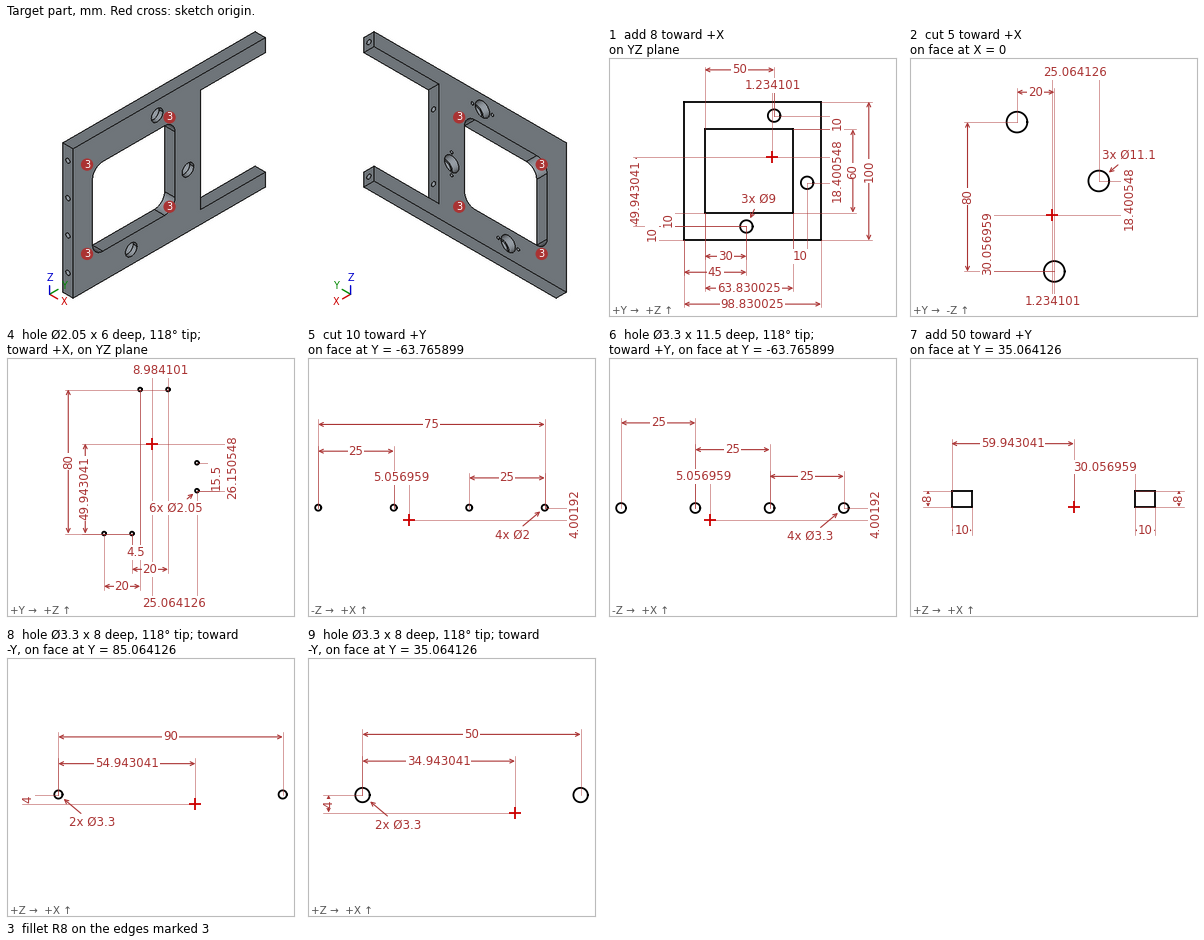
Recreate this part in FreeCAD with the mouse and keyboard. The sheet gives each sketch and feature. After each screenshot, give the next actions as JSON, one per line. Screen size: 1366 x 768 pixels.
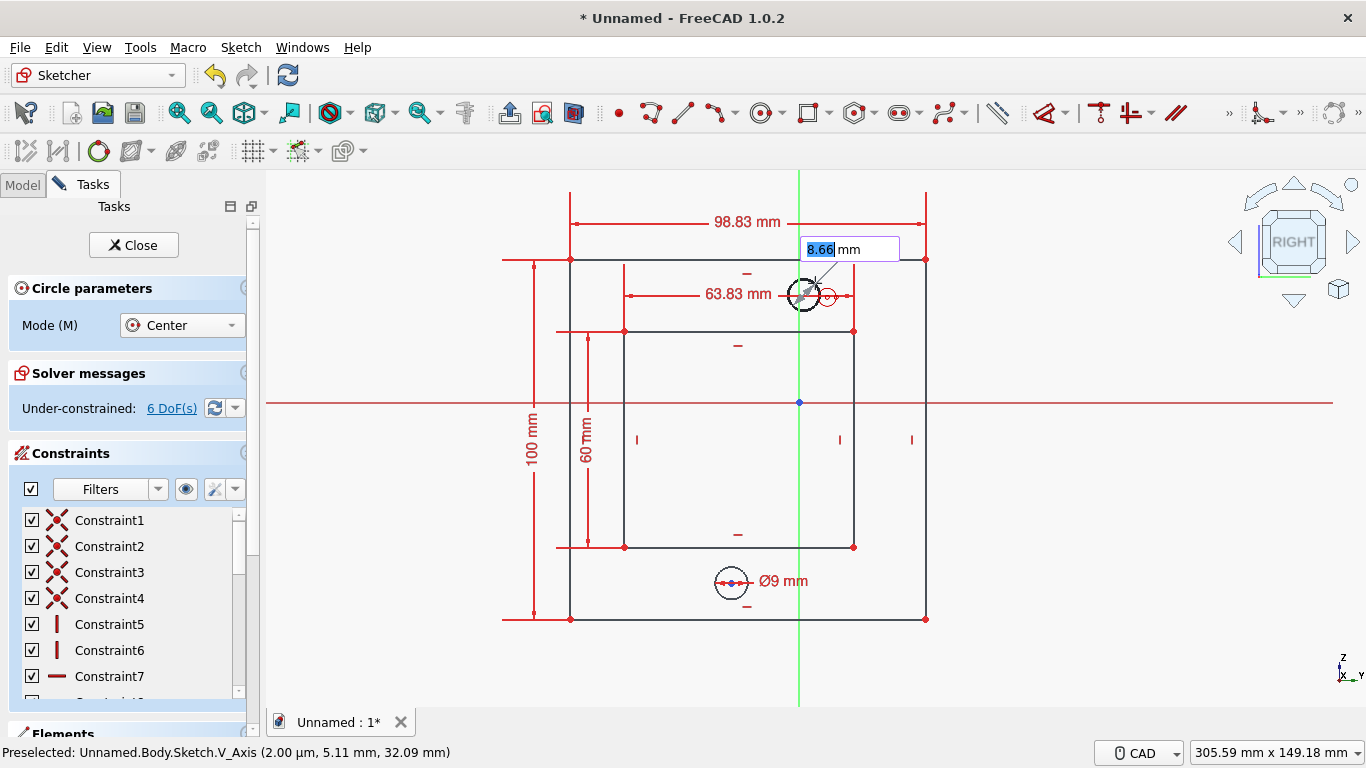
{"action": "type", "text": "9"}
{"action": "key", "text": "Return"}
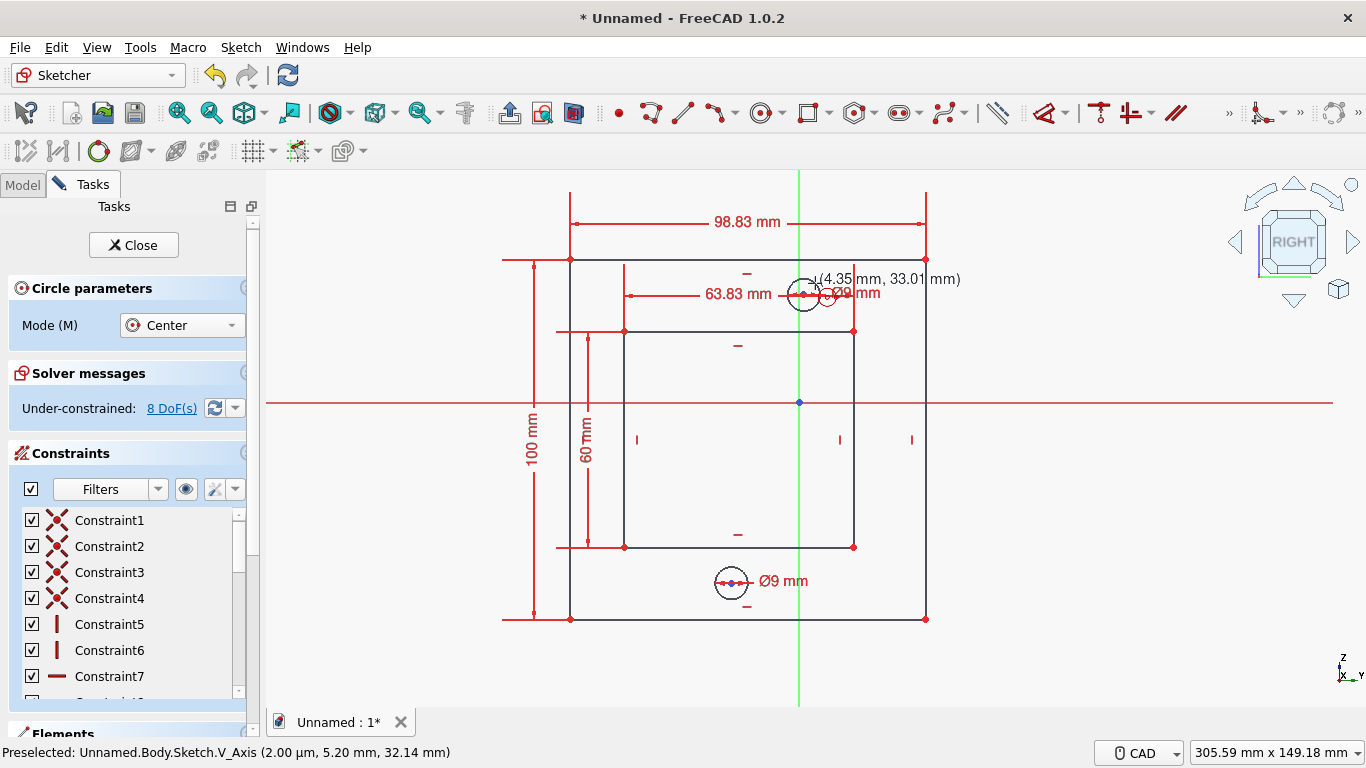
{"action": "scroll", "coordinate": [890, 469], "scroll_direction": "up", "scroll_amount": 2}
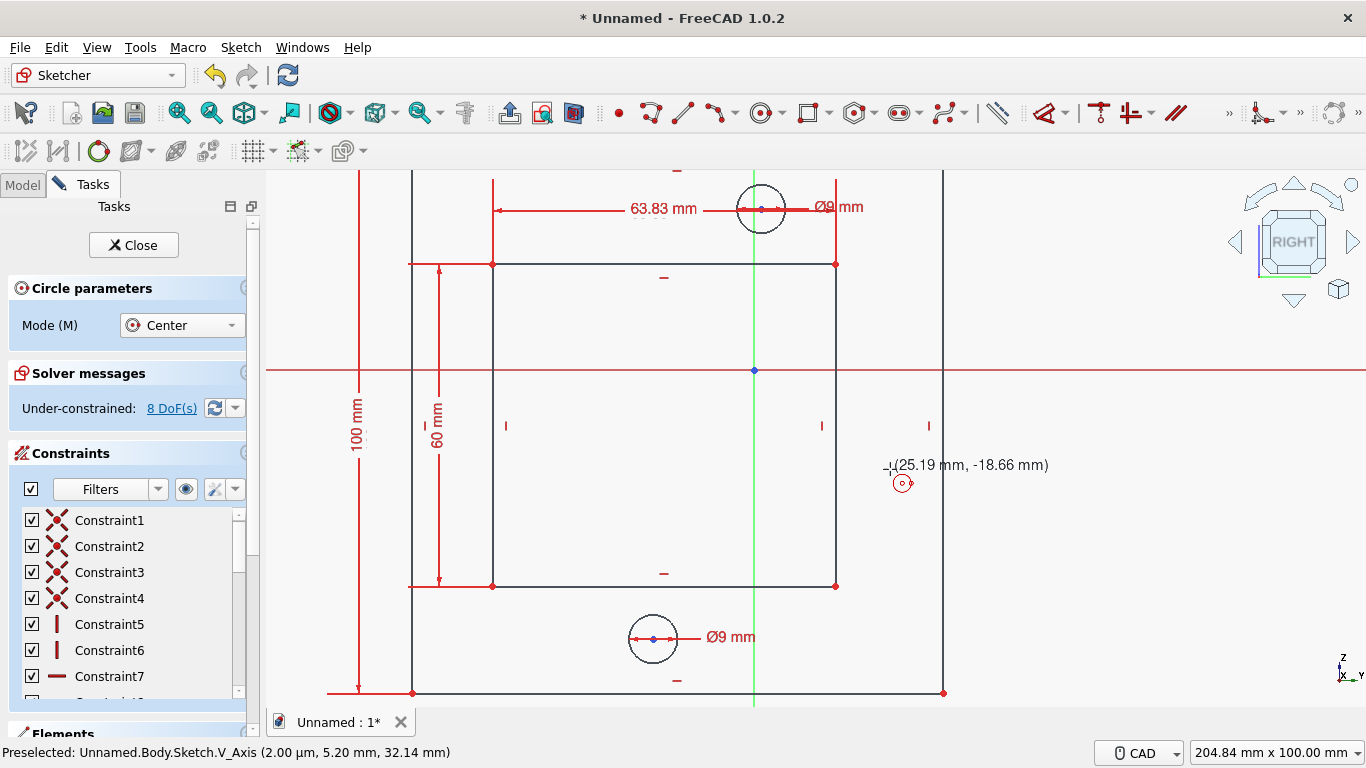
{"action": "left_click", "coordinate": [889, 469]}
{"action": "mouse_move", "coordinate": [906, 452]}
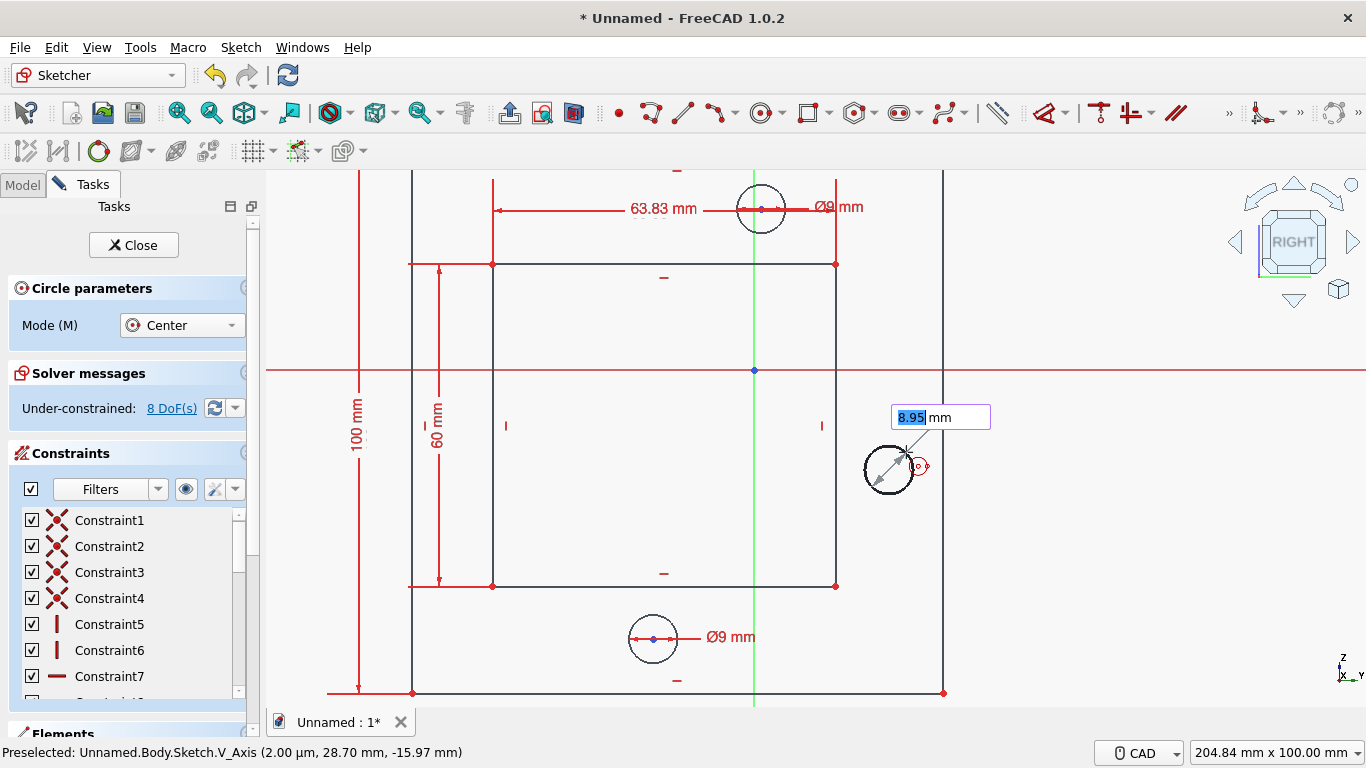
{"action": "type", "text": "9"}
{"action": "key", "text": "Return"}
{"action": "key", "text": "Escape"}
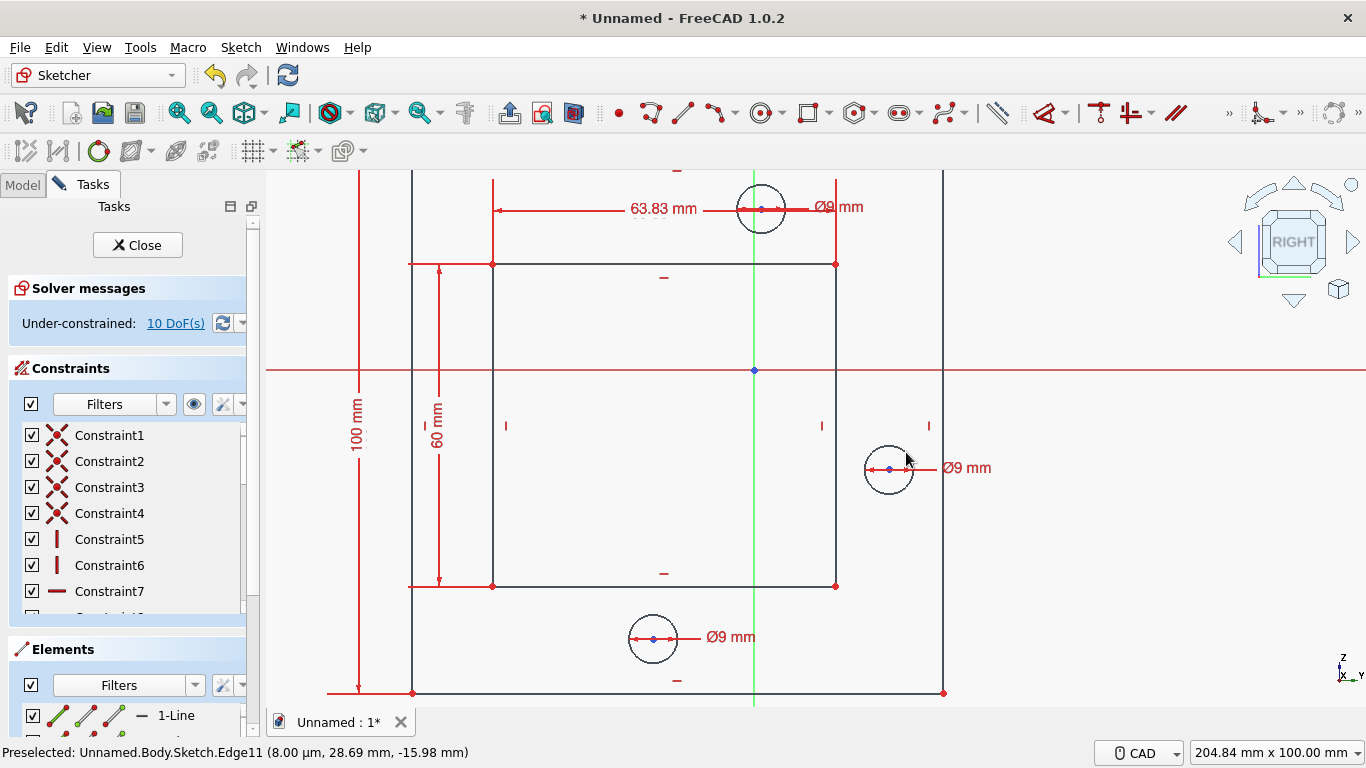
{"action": "left_click", "coordinate": [493, 587]}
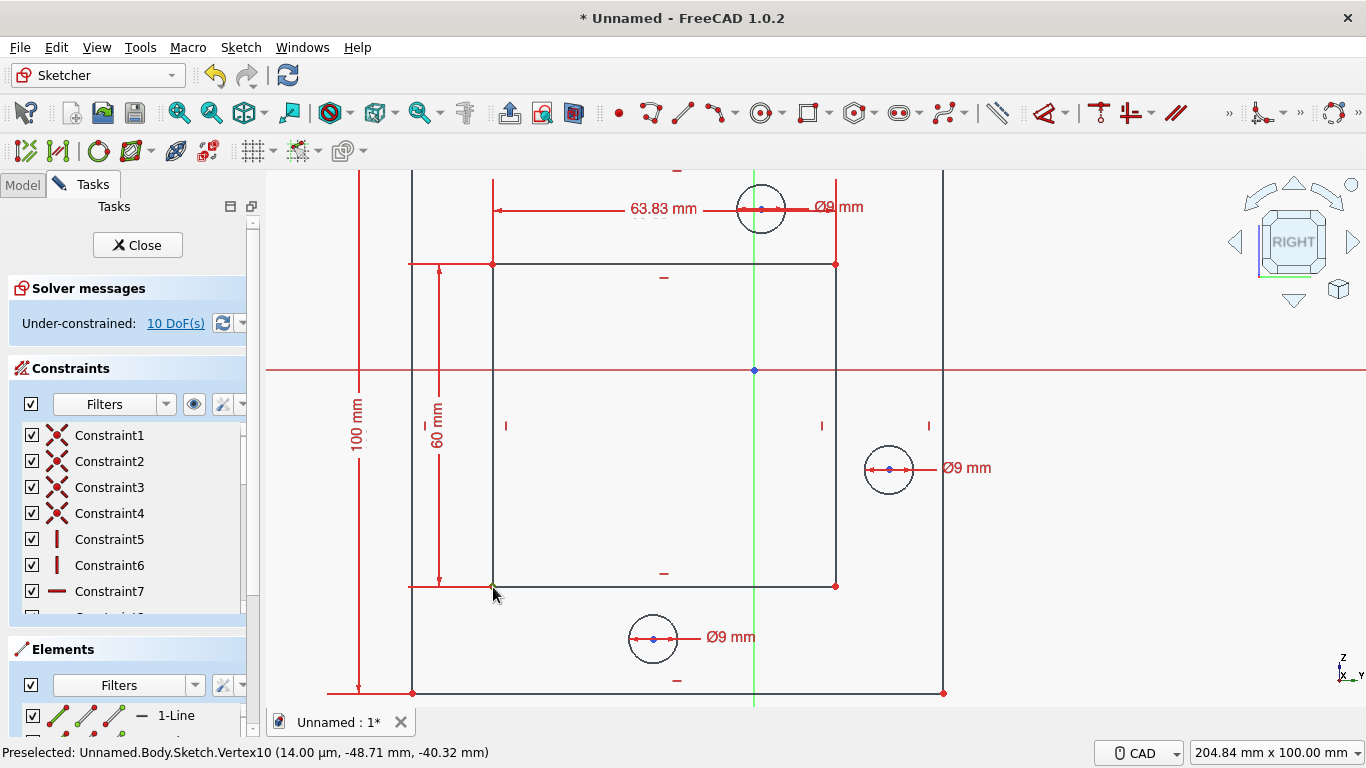
{"action": "left_click", "coordinate": [653, 639]}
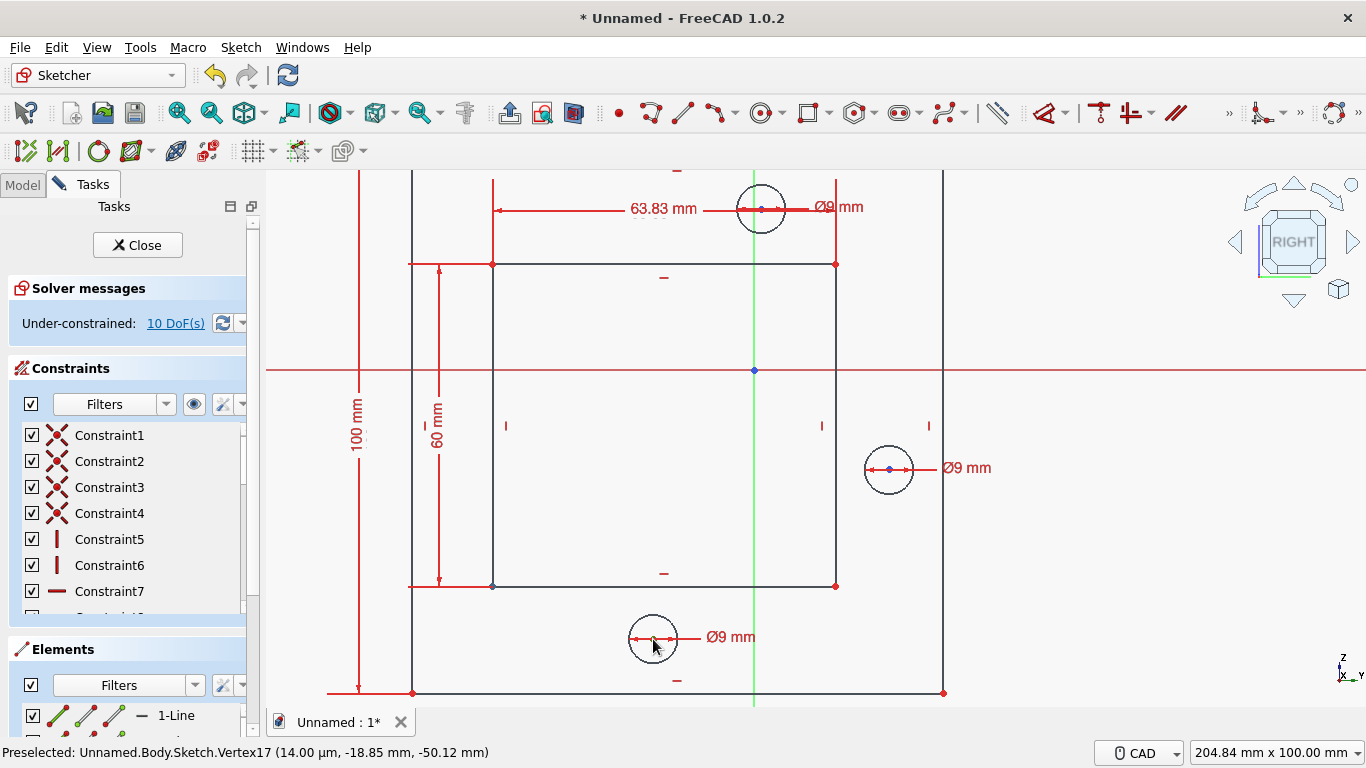
{"action": "key", "text": "l"}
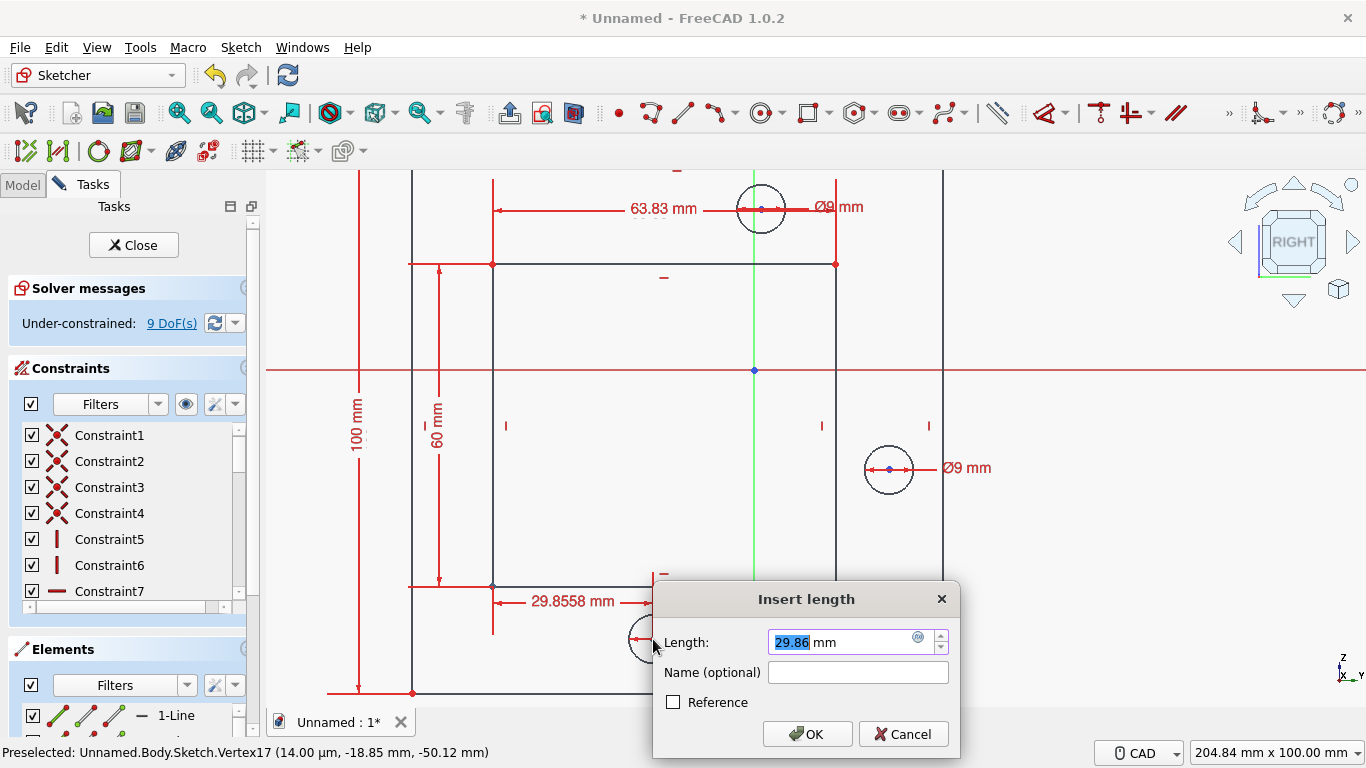
{"action": "type", "text": "30"}
{"action": "key", "text": "Return"}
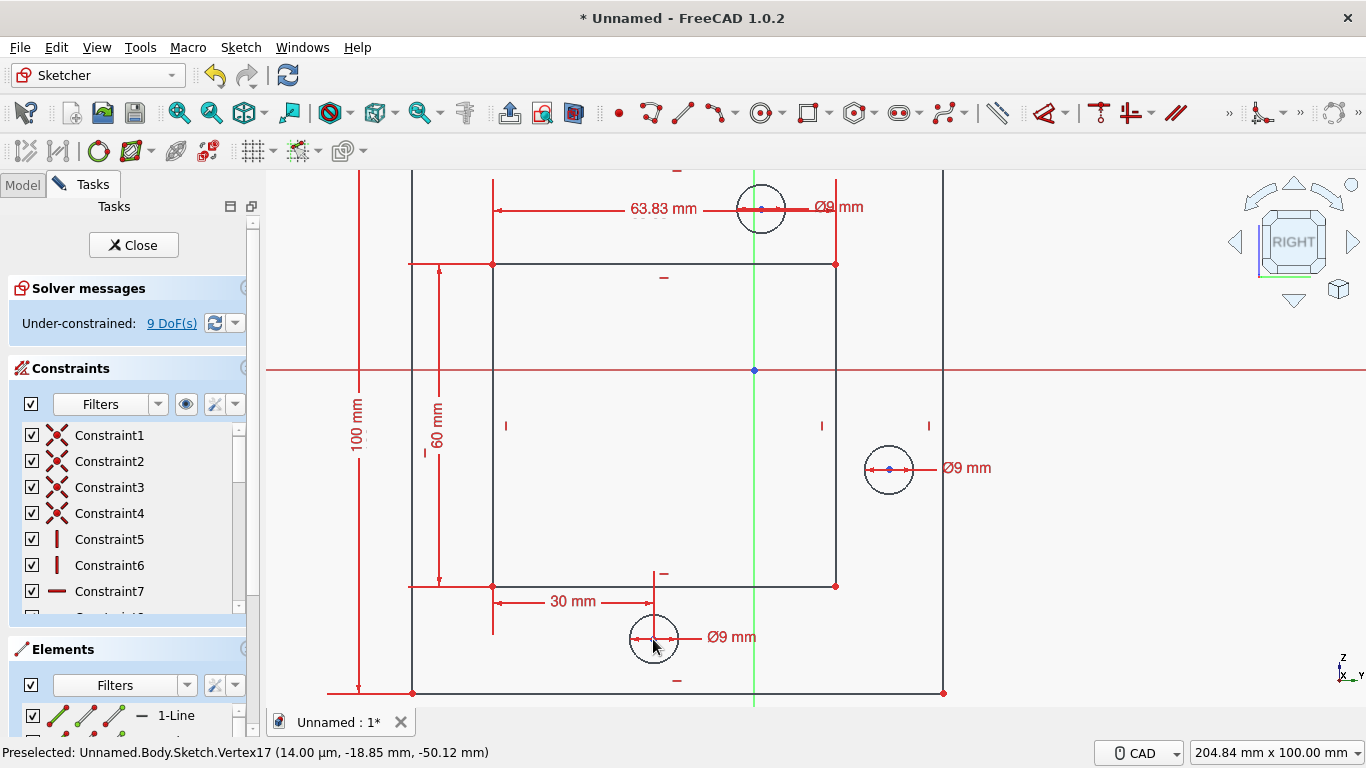
{"action": "scroll", "coordinate": [890, 469], "scroll_direction": "down", "scroll_amount": 2}